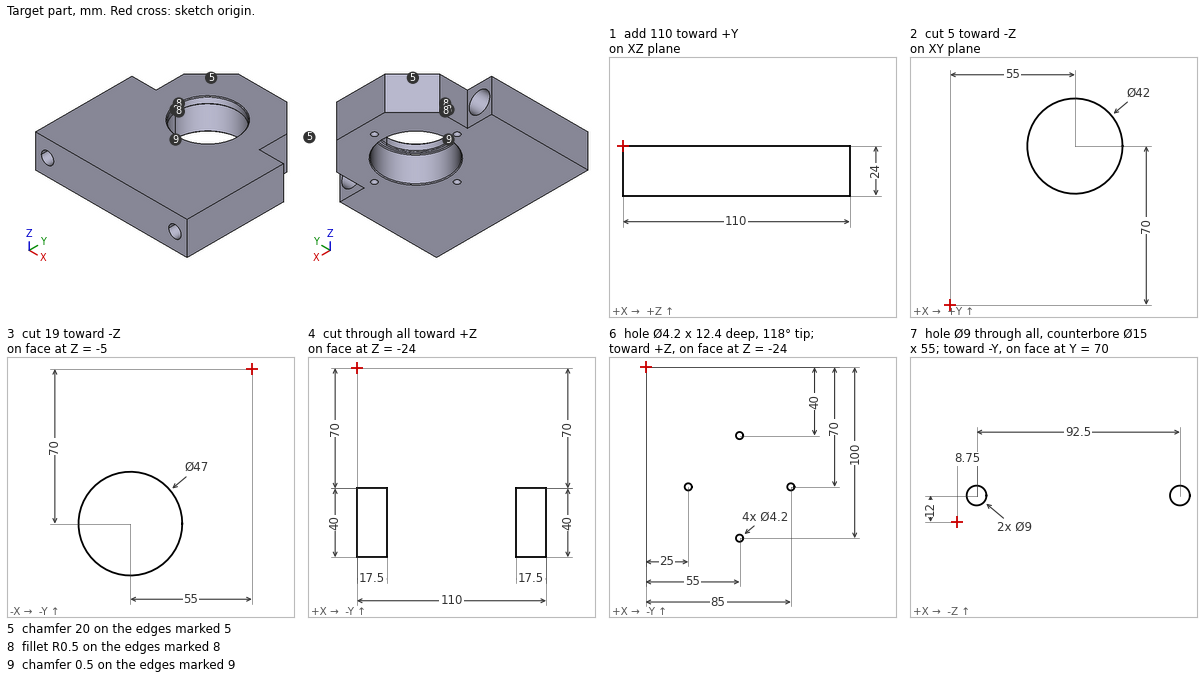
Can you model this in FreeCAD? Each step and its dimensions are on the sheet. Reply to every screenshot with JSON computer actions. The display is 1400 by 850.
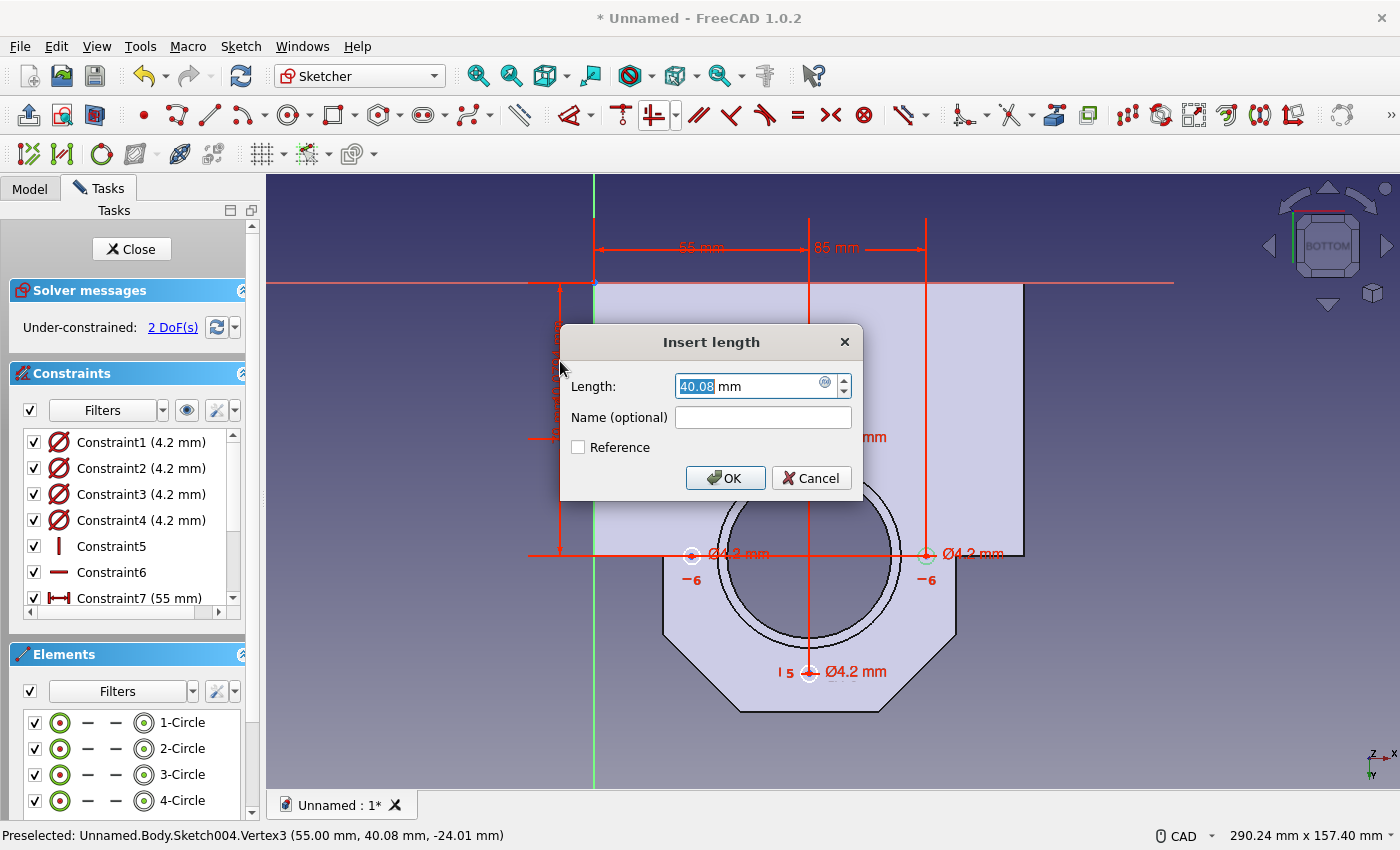
{"action": "type", "text": "40"}
{"action": "key", "text": "Return"}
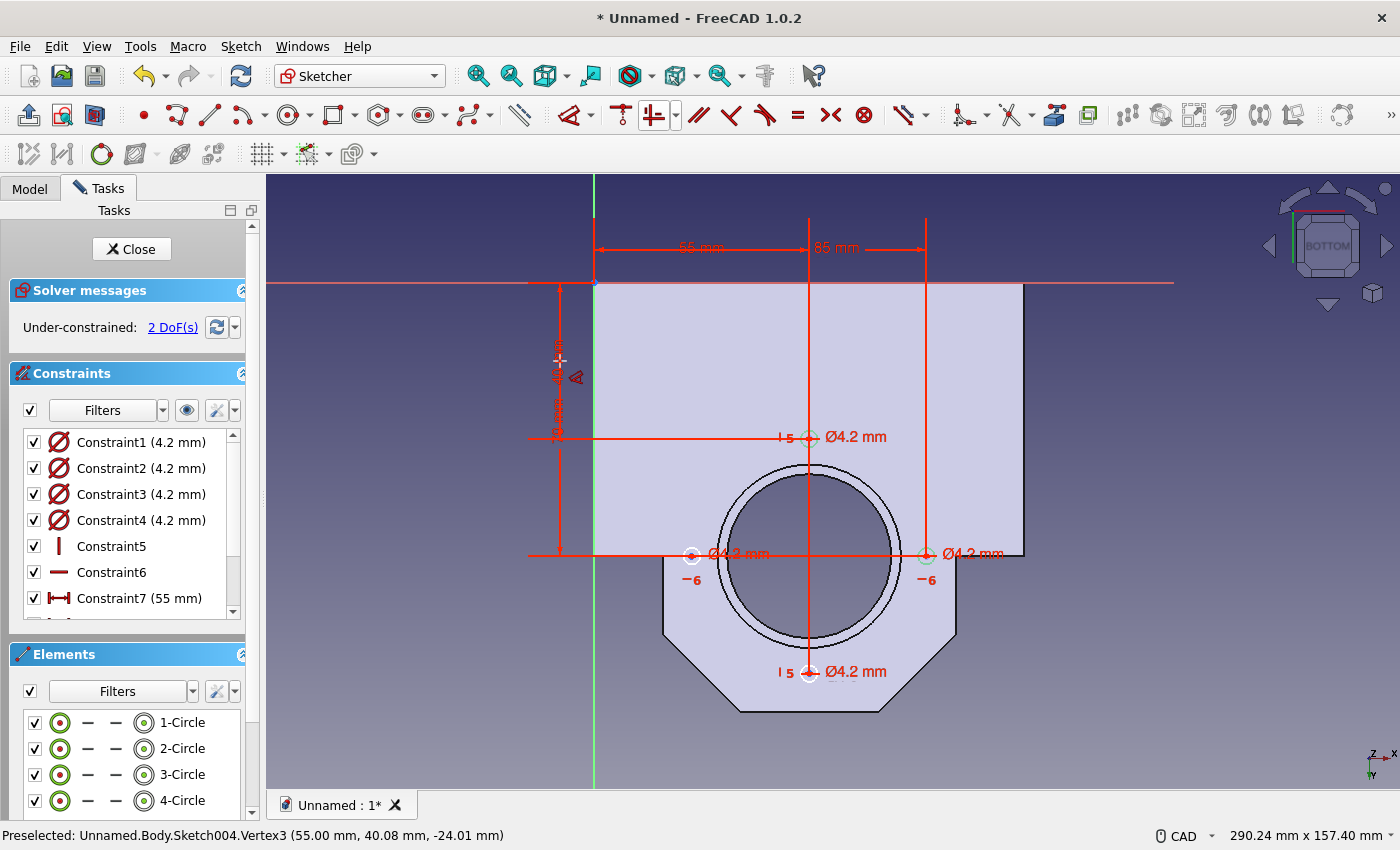
{"action": "left_click", "coordinate": [692, 556]}
{"action": "left_click", "coordinate": [621, 249]}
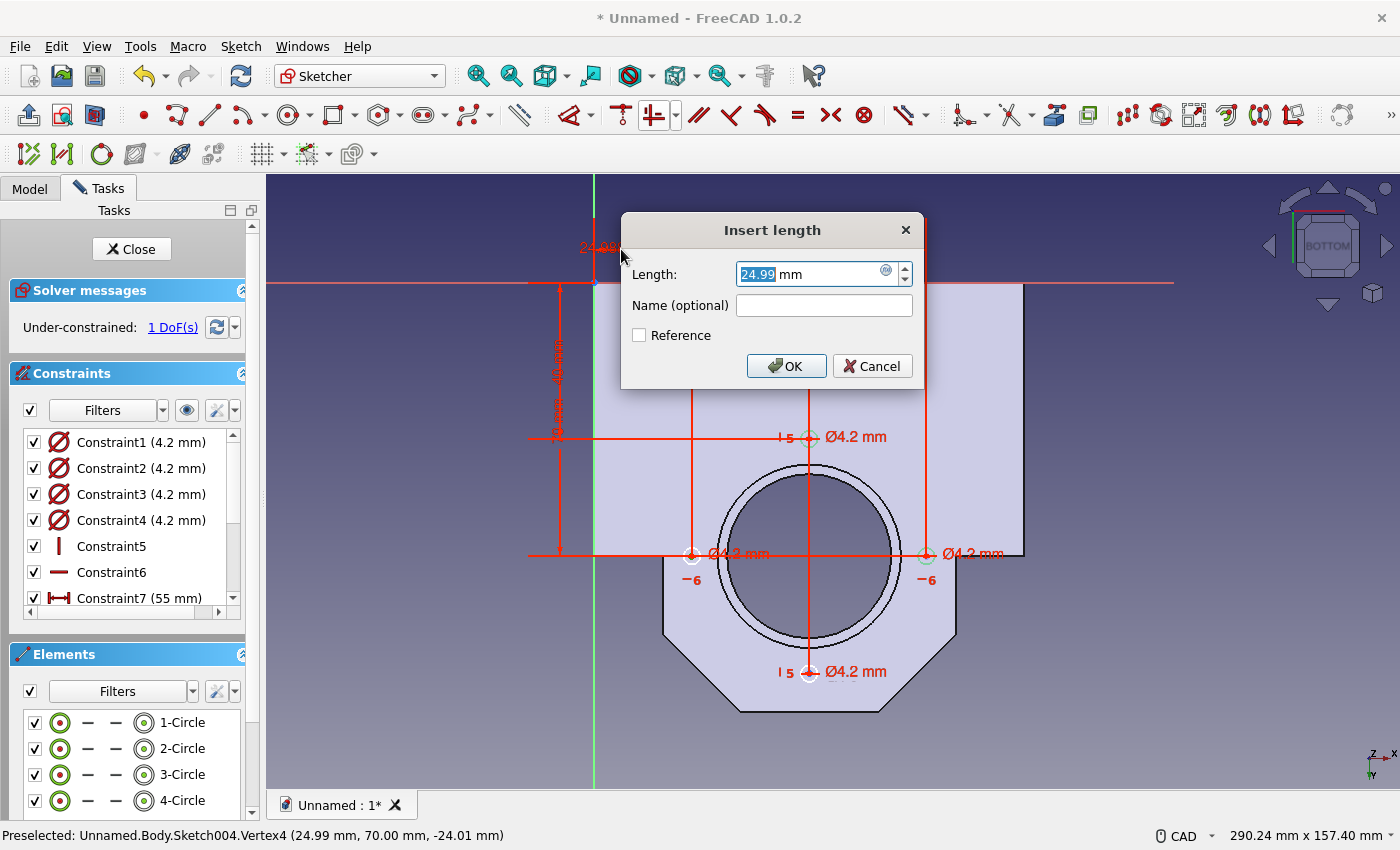
{"action": "type", "text": "25"}
{"action": "key", "text": "Return"}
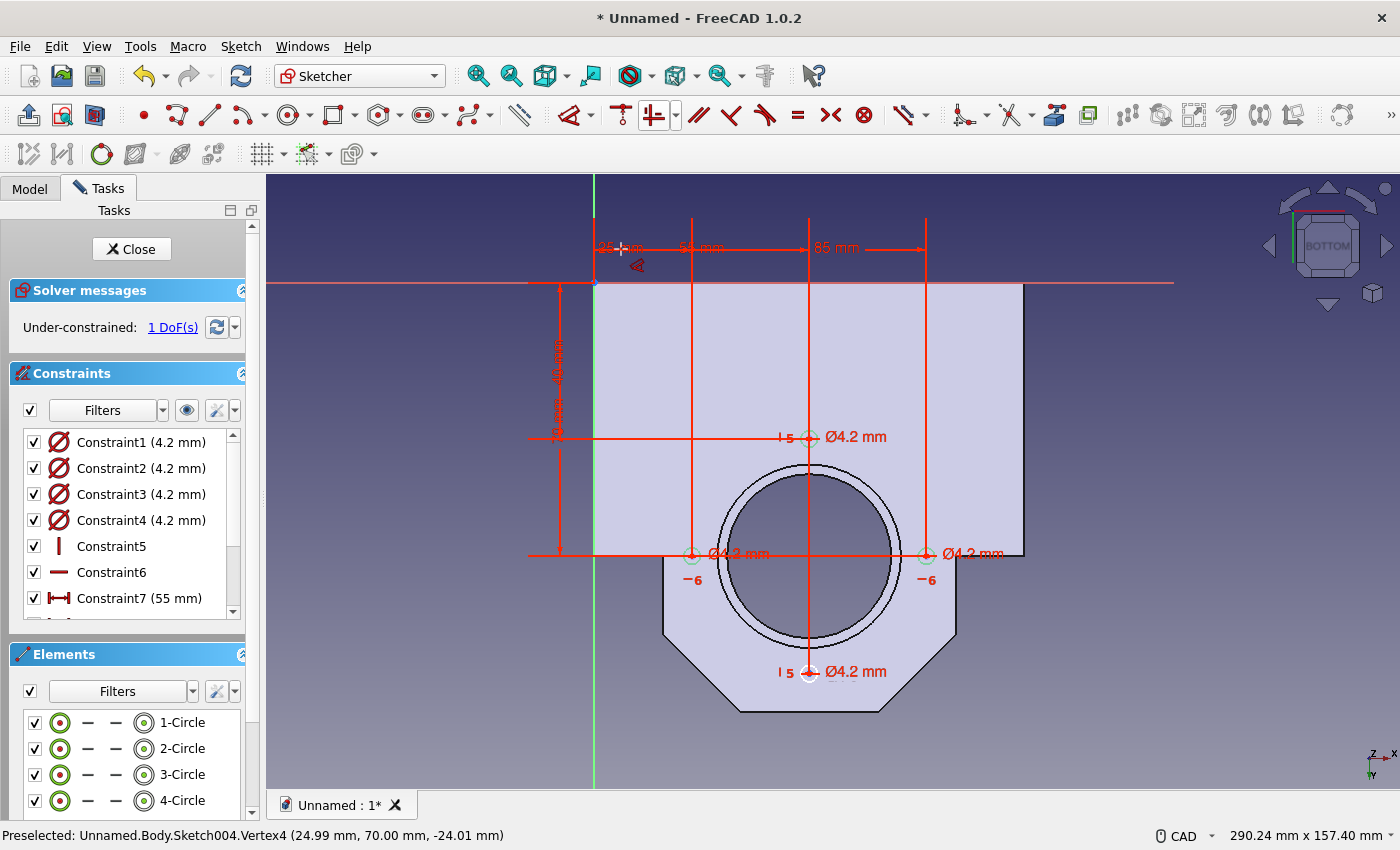
{"action": "left_click", "coordinate": [809, 674]}
{"action": "left_click", "coordinate": [560, 478]}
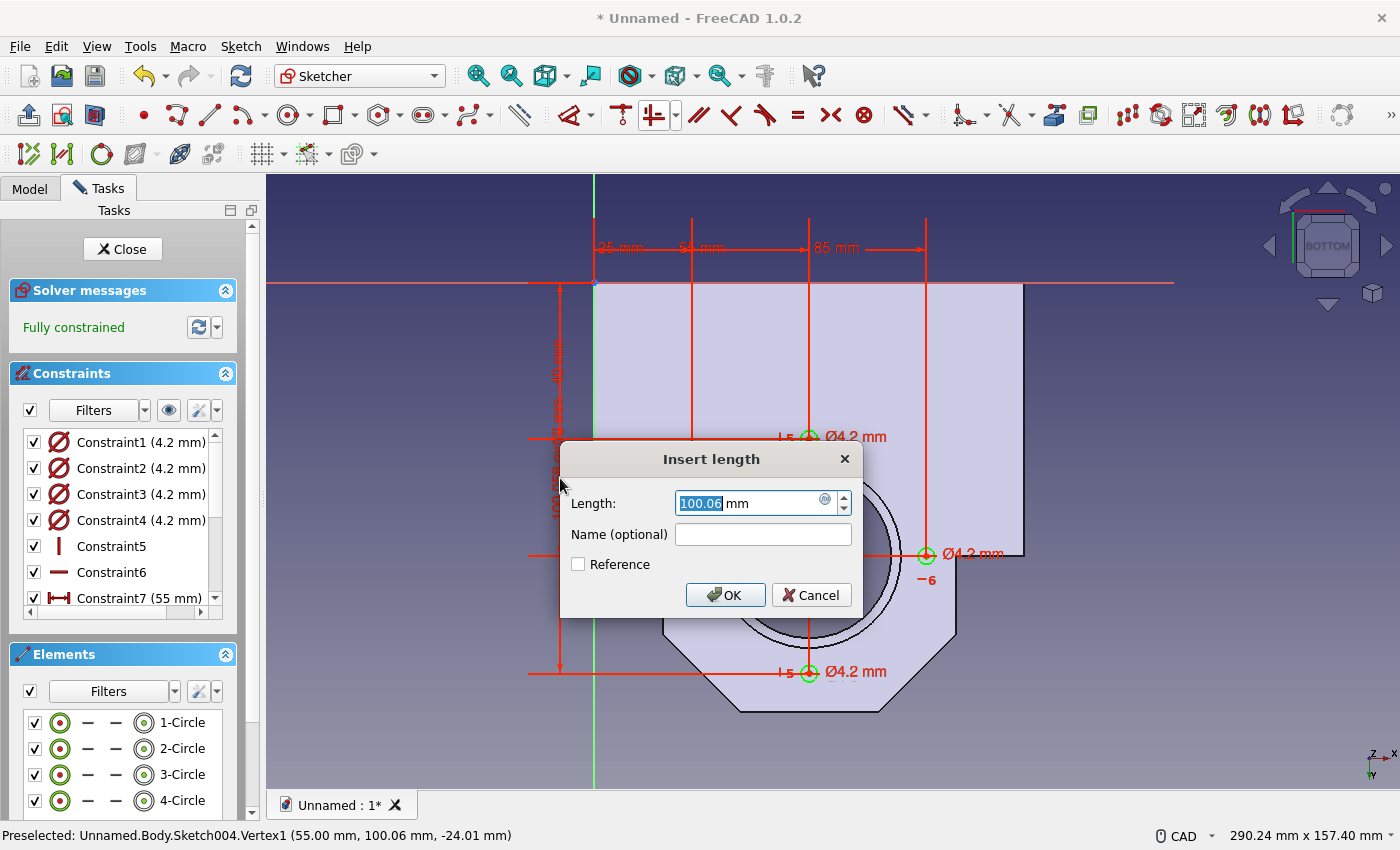
{"action": "type", "text": "100"}
{"action": "key", "text": "Return"}
{"action": "key", "text": "Escape"}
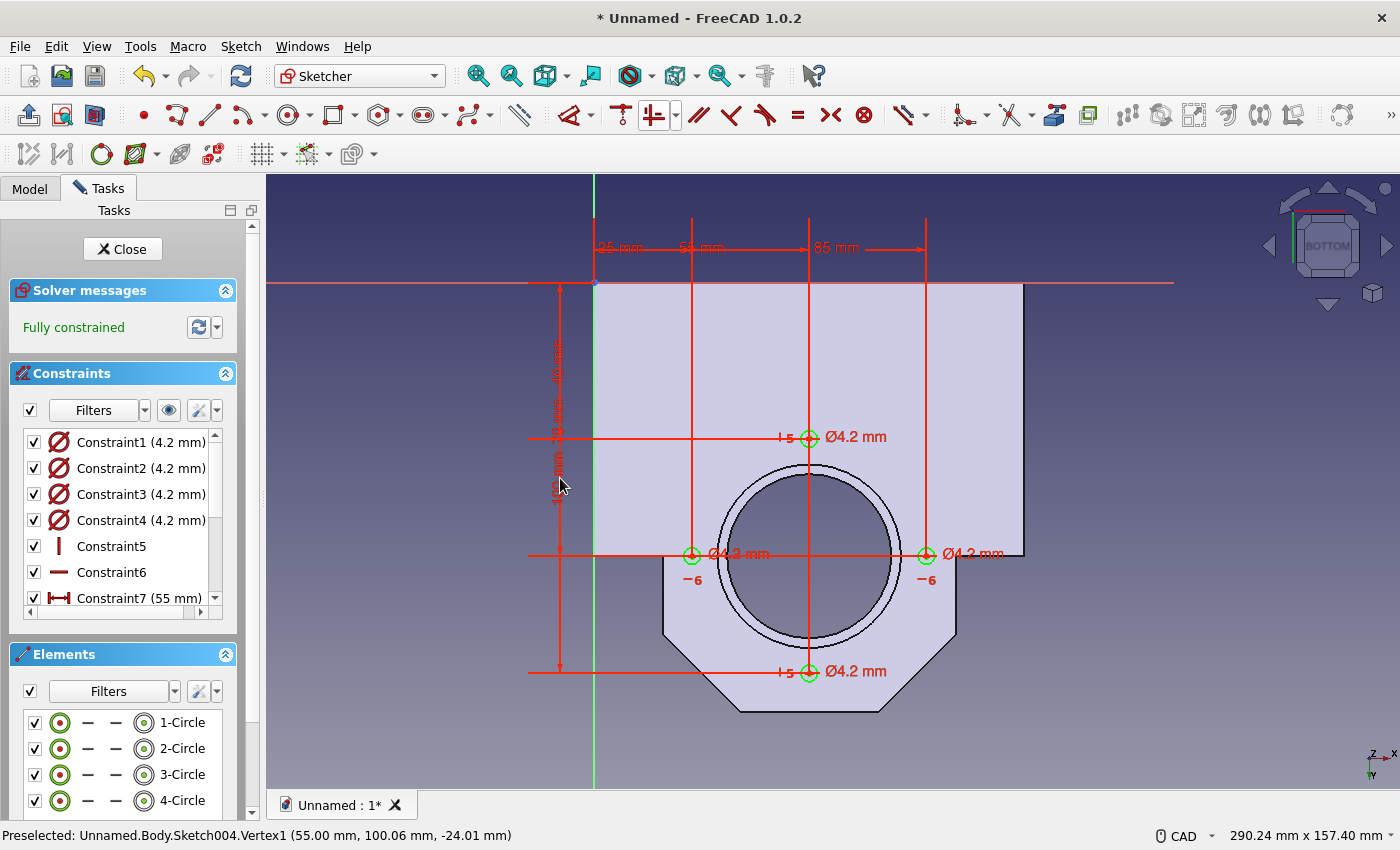
{"action": "left_click", "coordinate": [123, 249]}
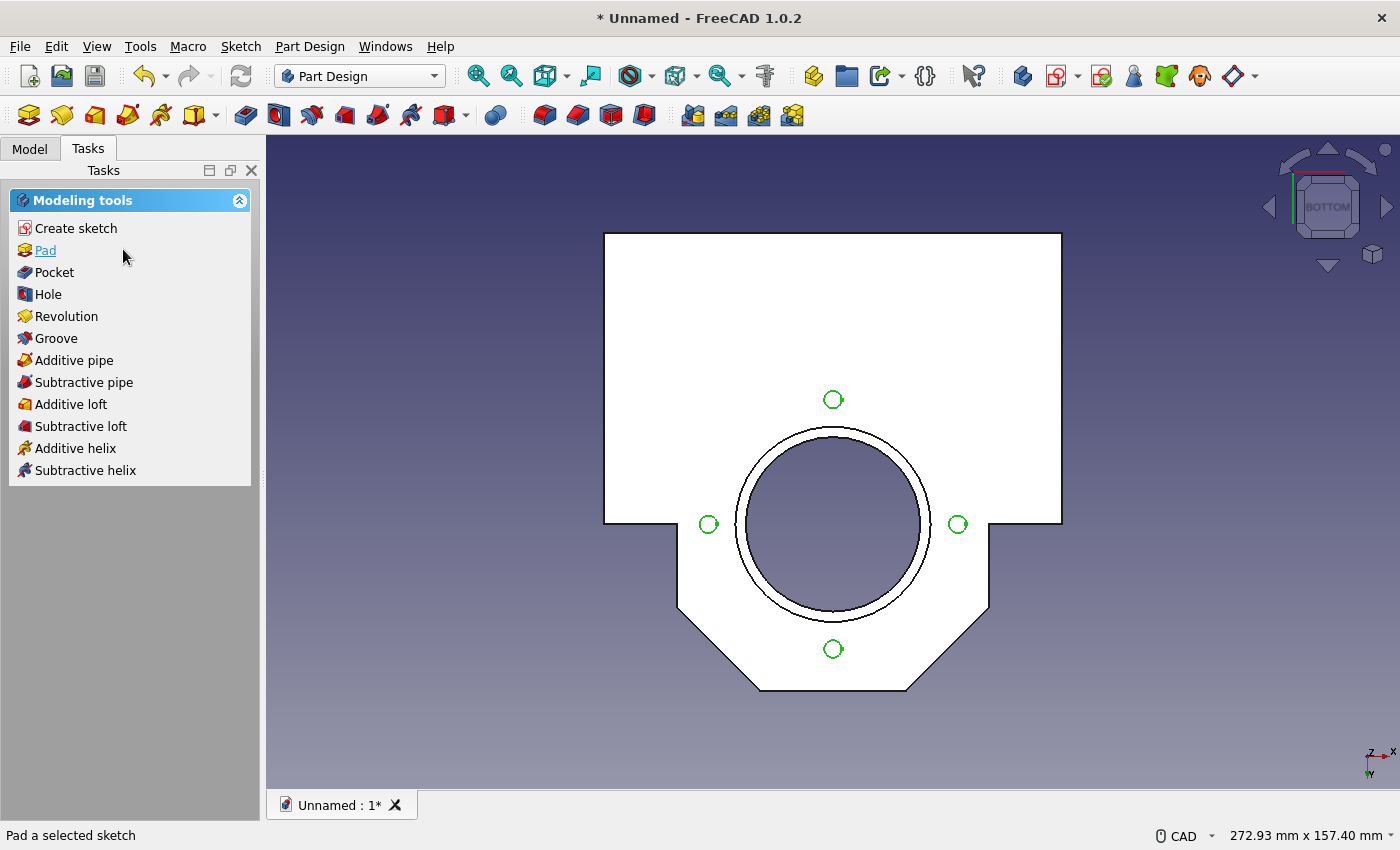
{"action": "left_click", "coordinate": [279, 116]}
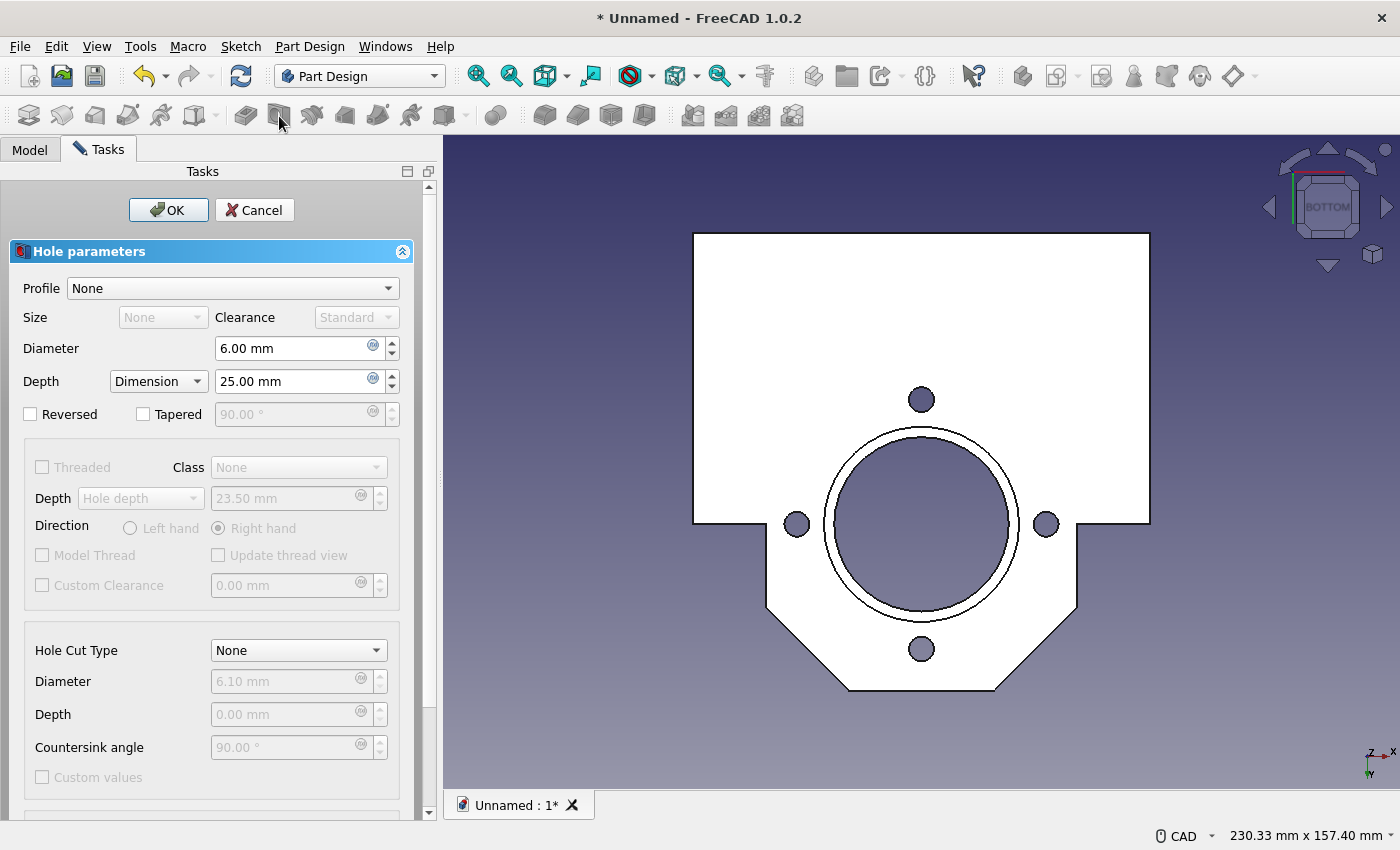
{"action": "triple_click", "coordinate": [300, 348]}